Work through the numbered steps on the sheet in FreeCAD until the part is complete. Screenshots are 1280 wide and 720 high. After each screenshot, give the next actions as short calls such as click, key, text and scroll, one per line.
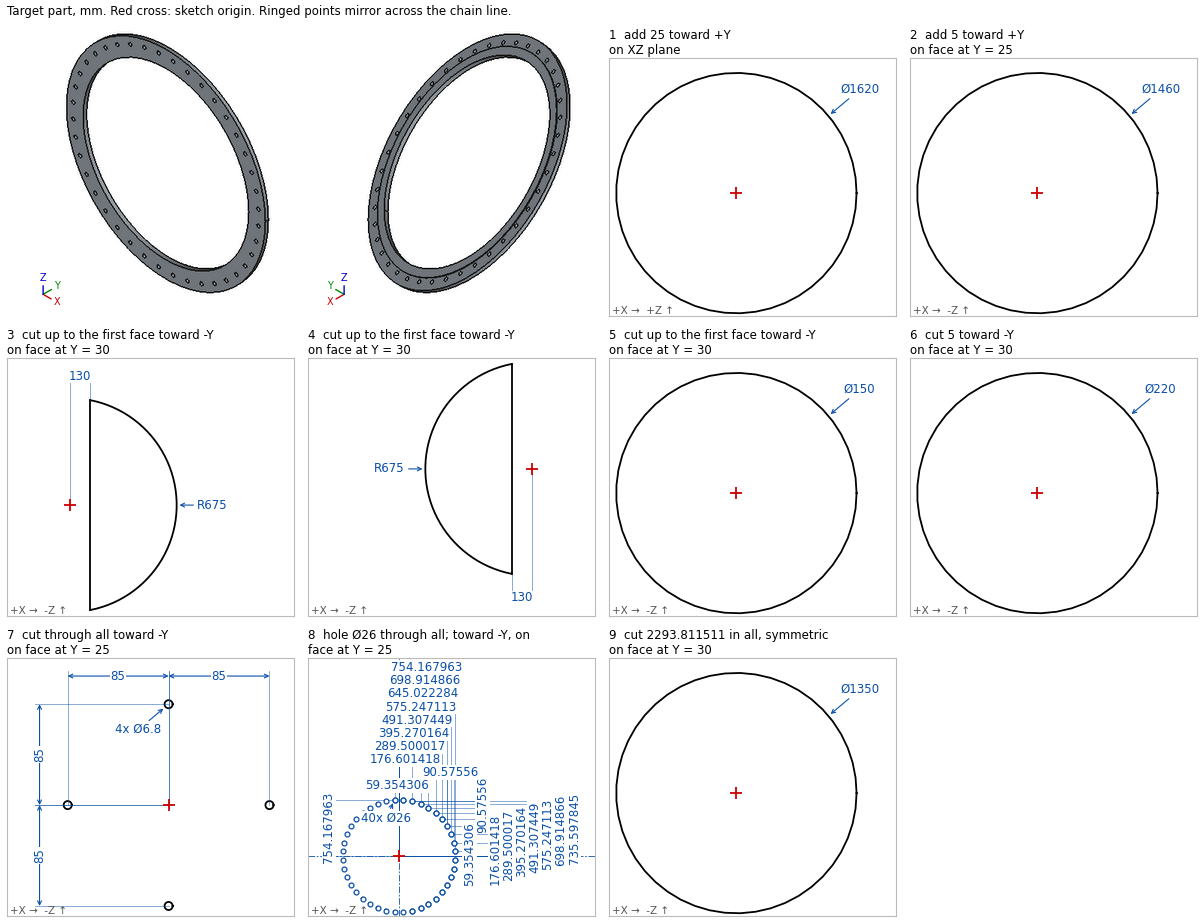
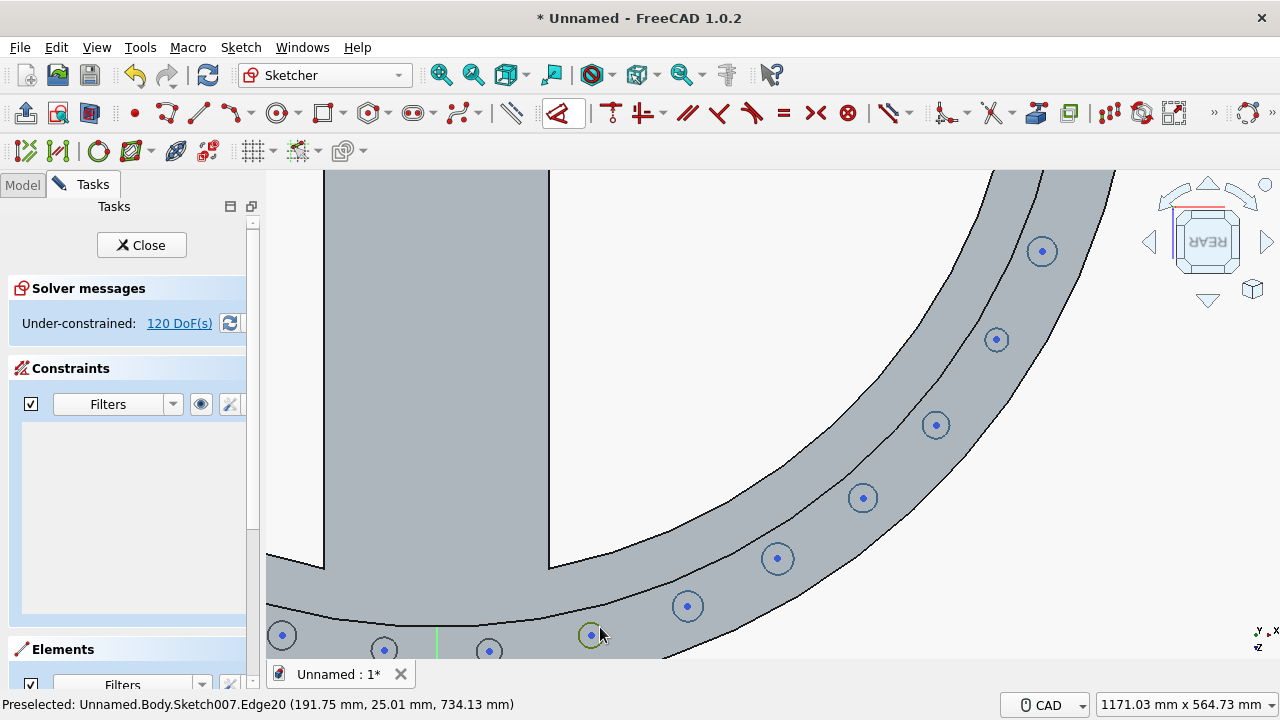
scroll(792, 552, down, 7)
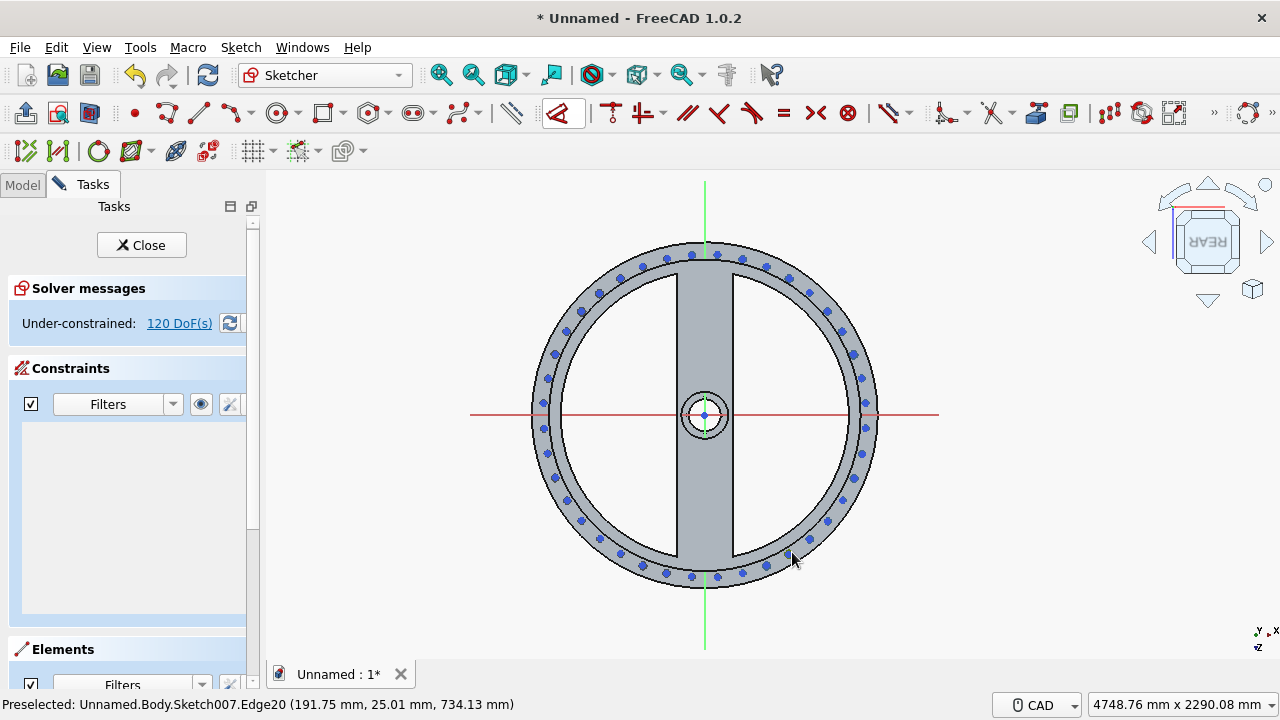
scroll(720, 575, up, 8)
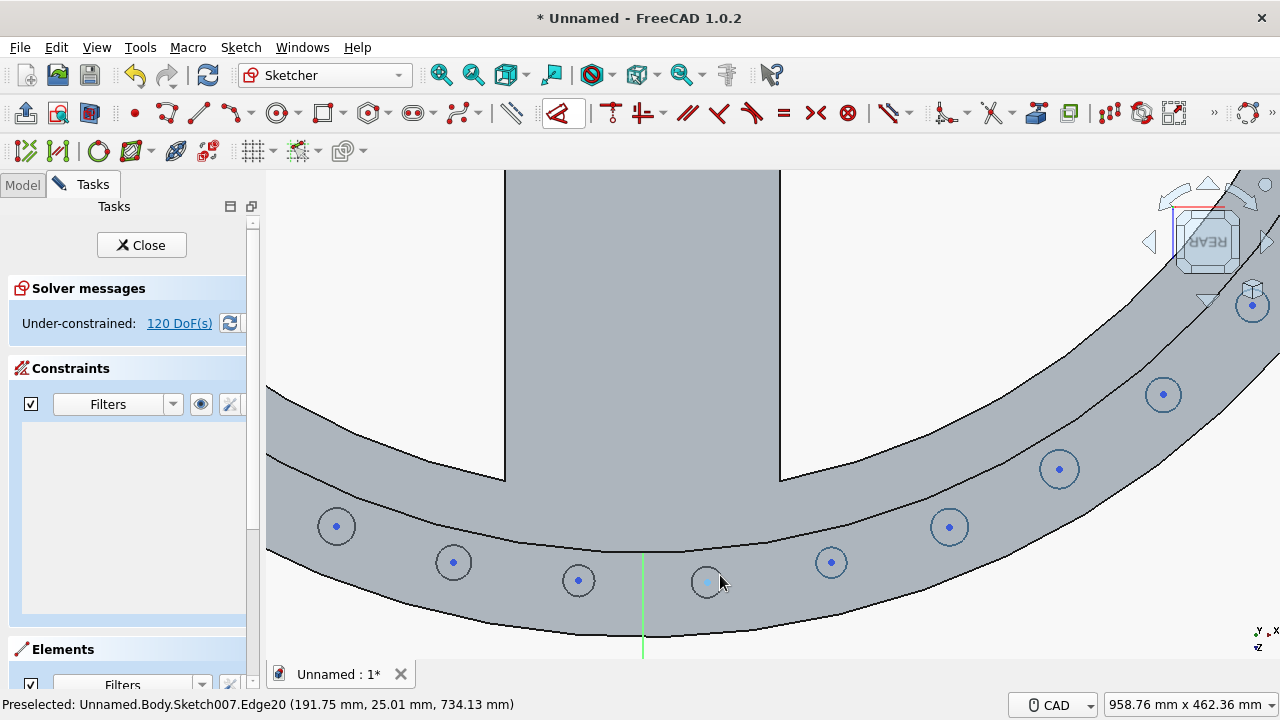
click(718, 571)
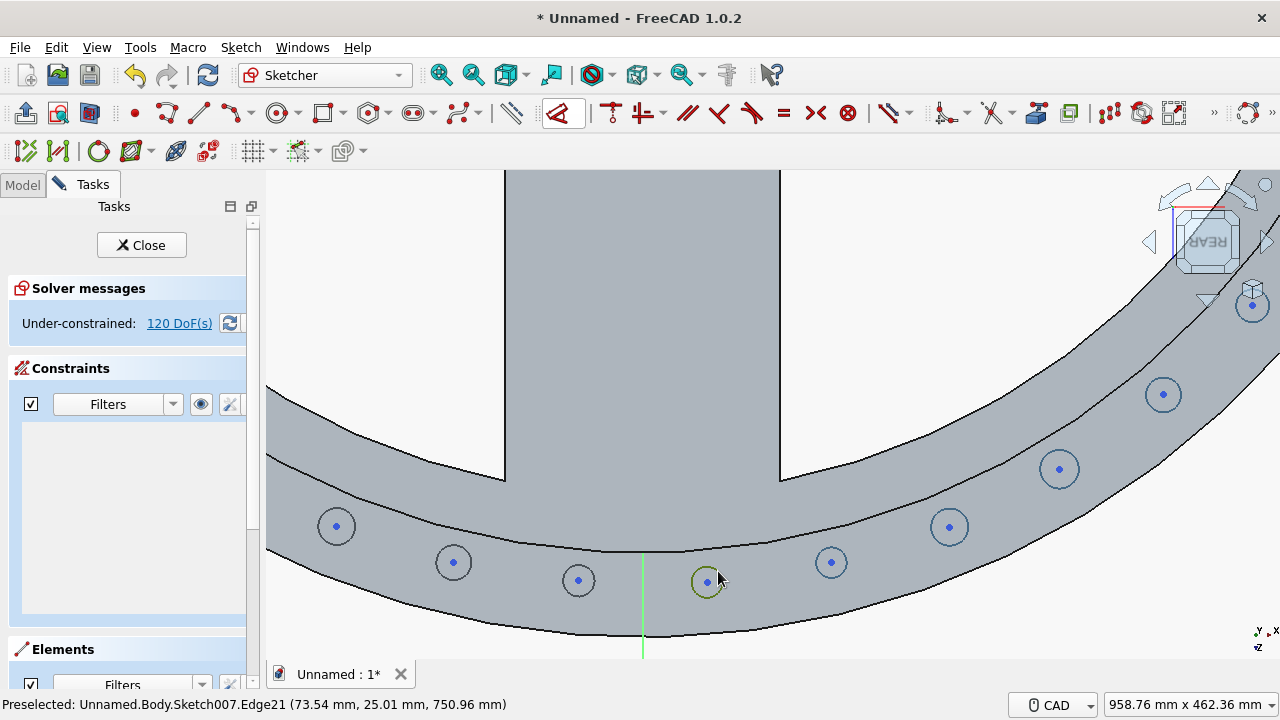
click(590, 570)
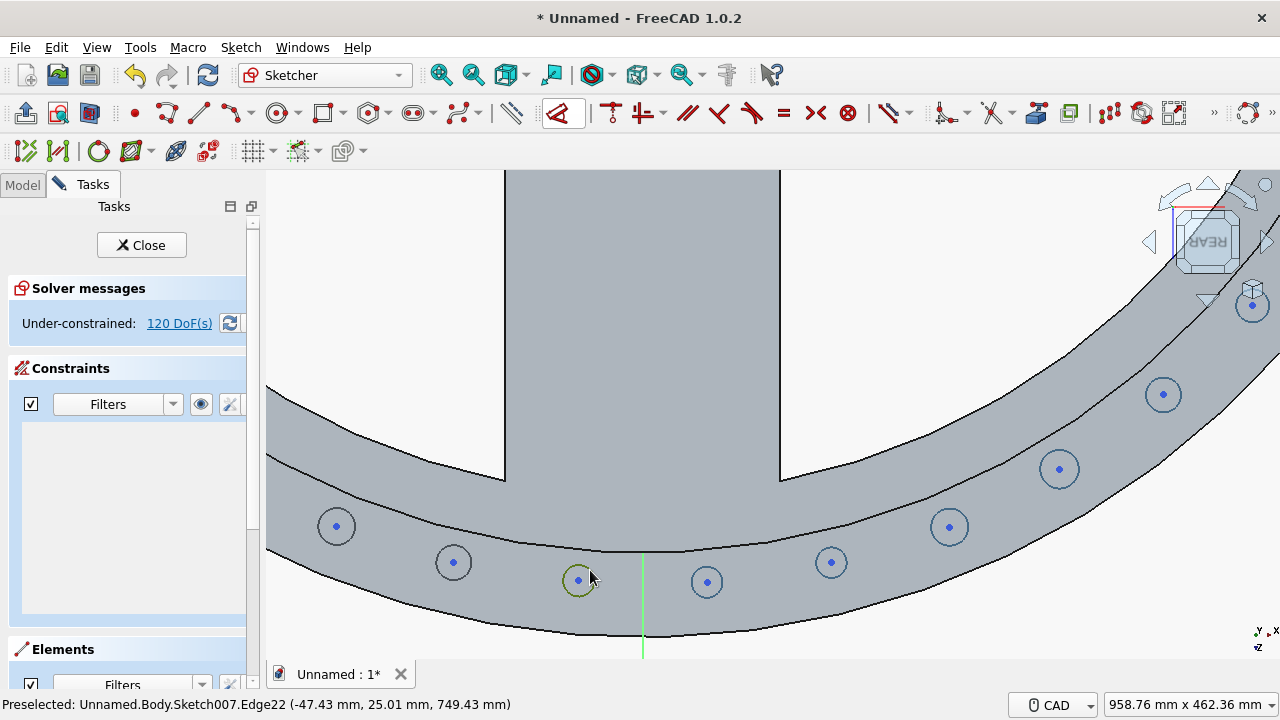
click(466, 550)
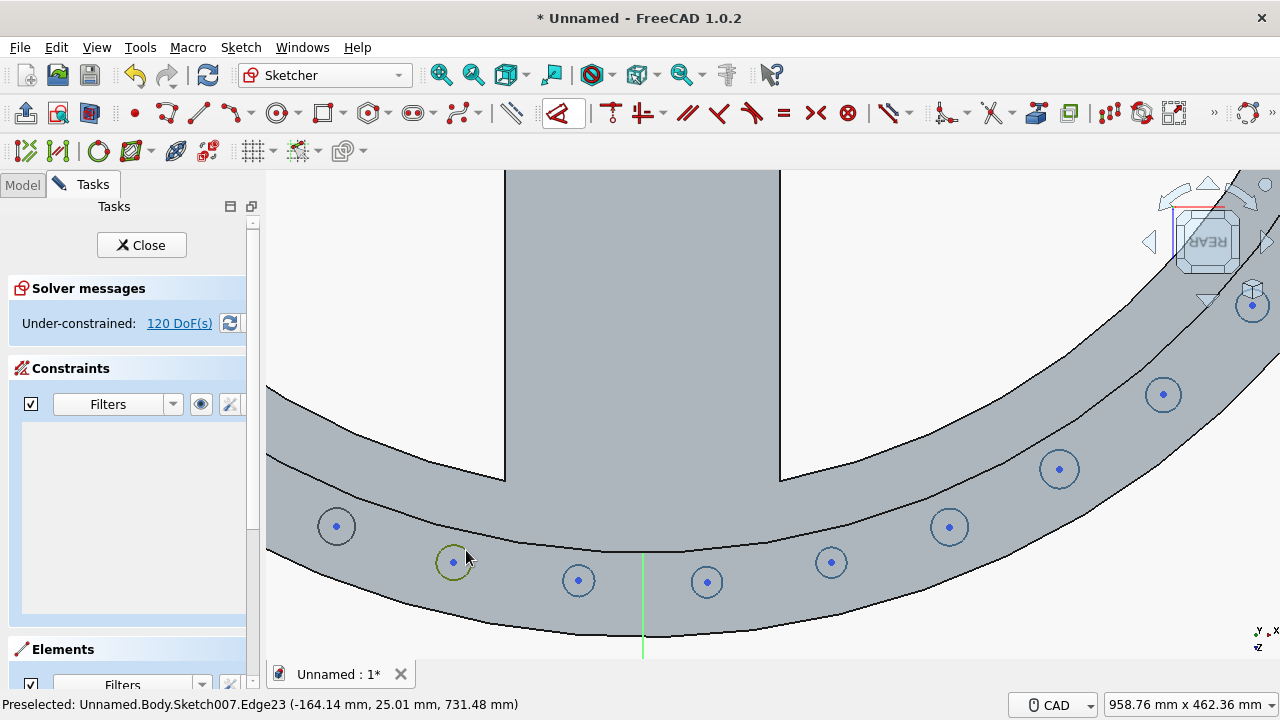
click(350, 513)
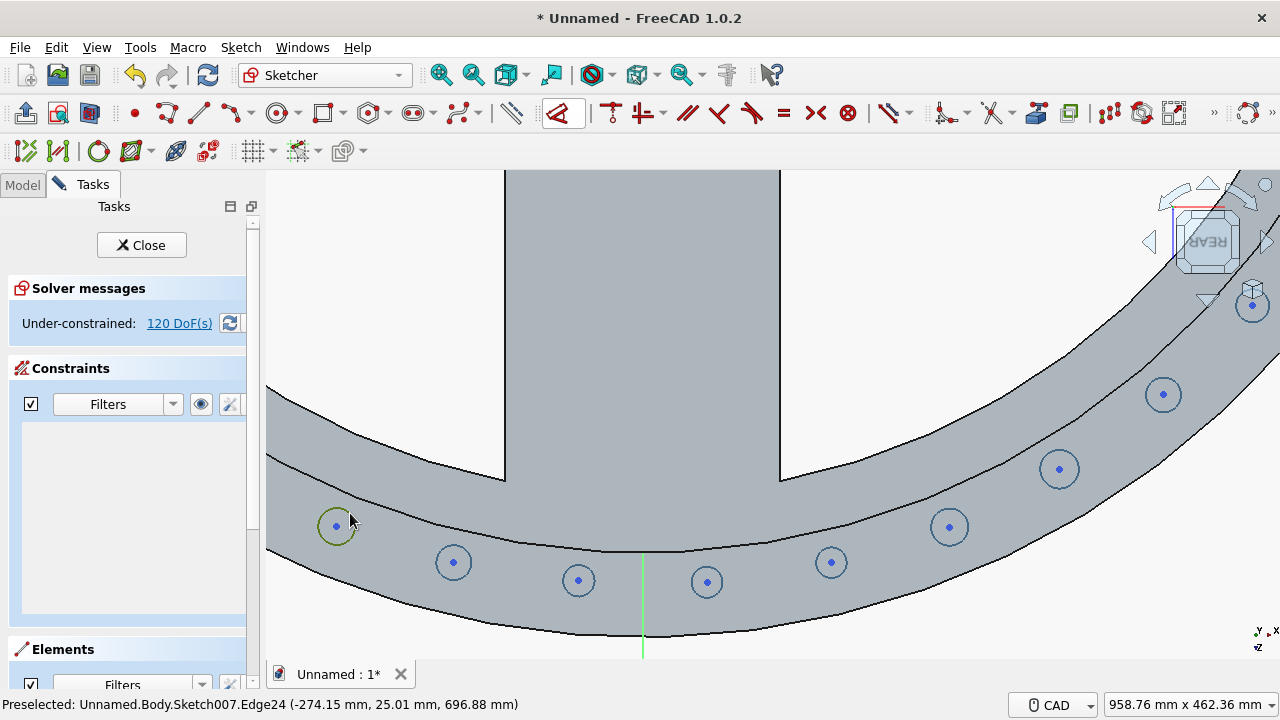
scroll(720, 575, down, 8)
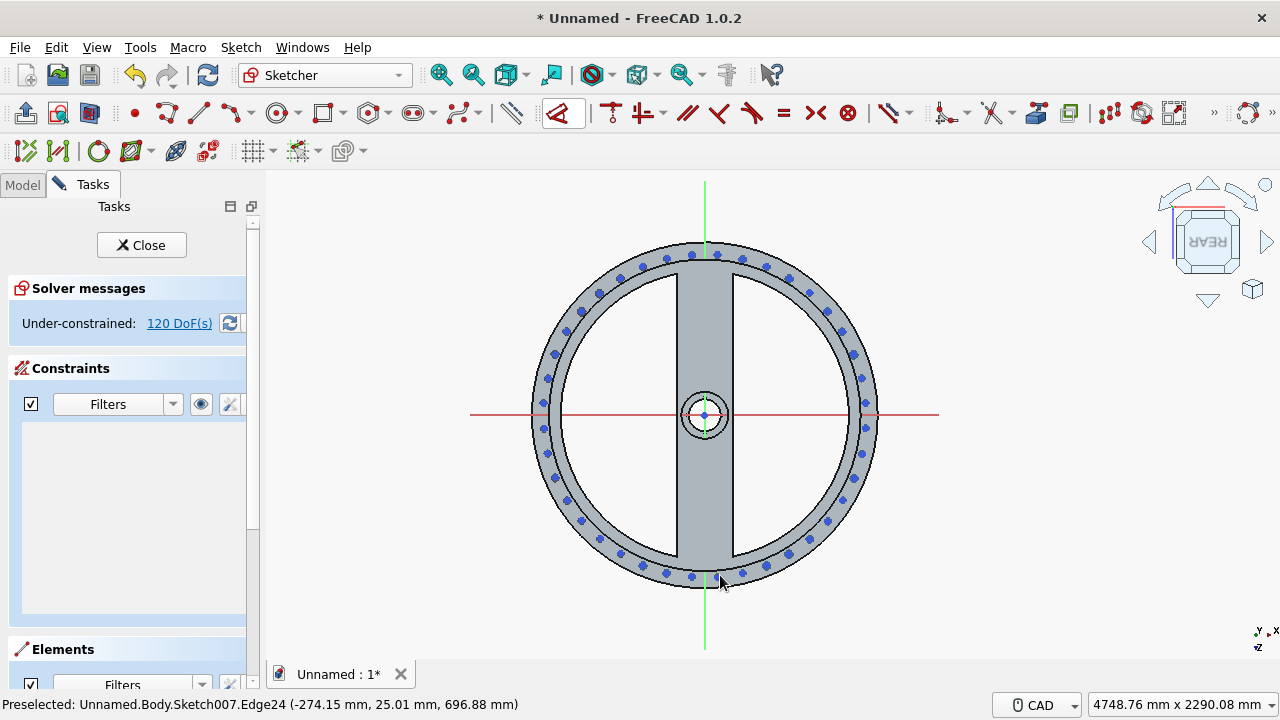
scroll(623, 552, up, 8)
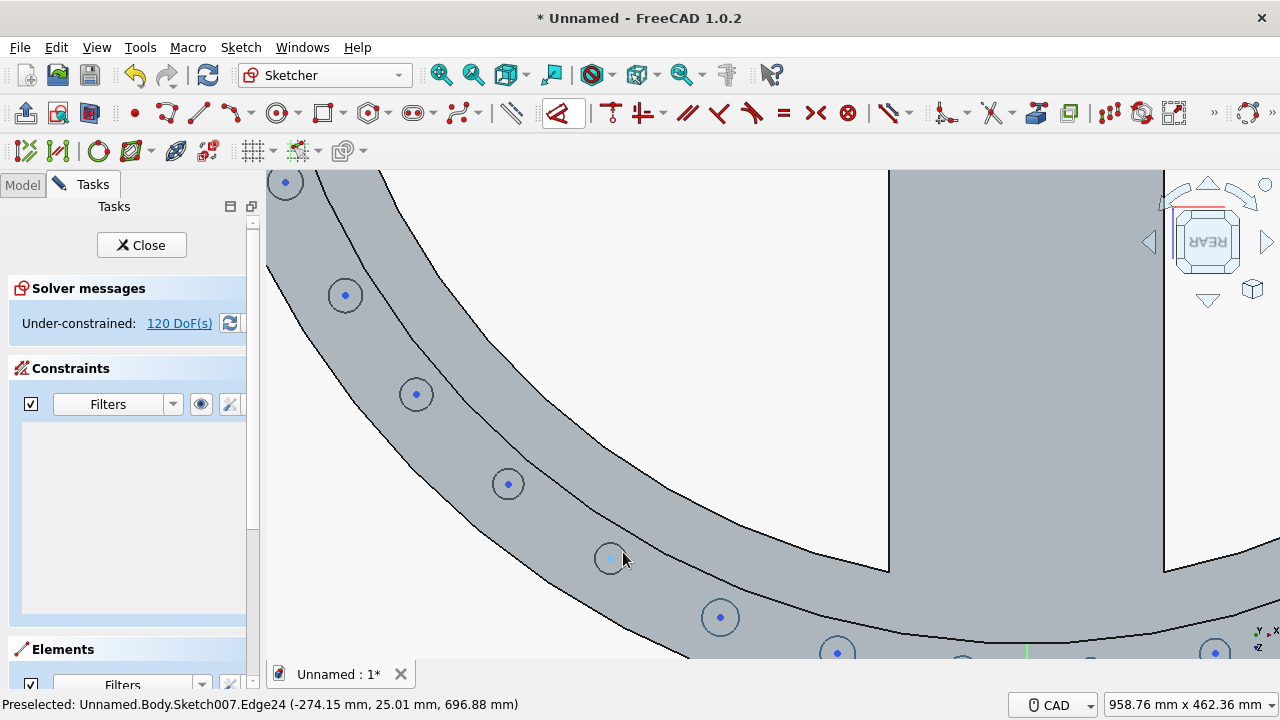
click(621, 548)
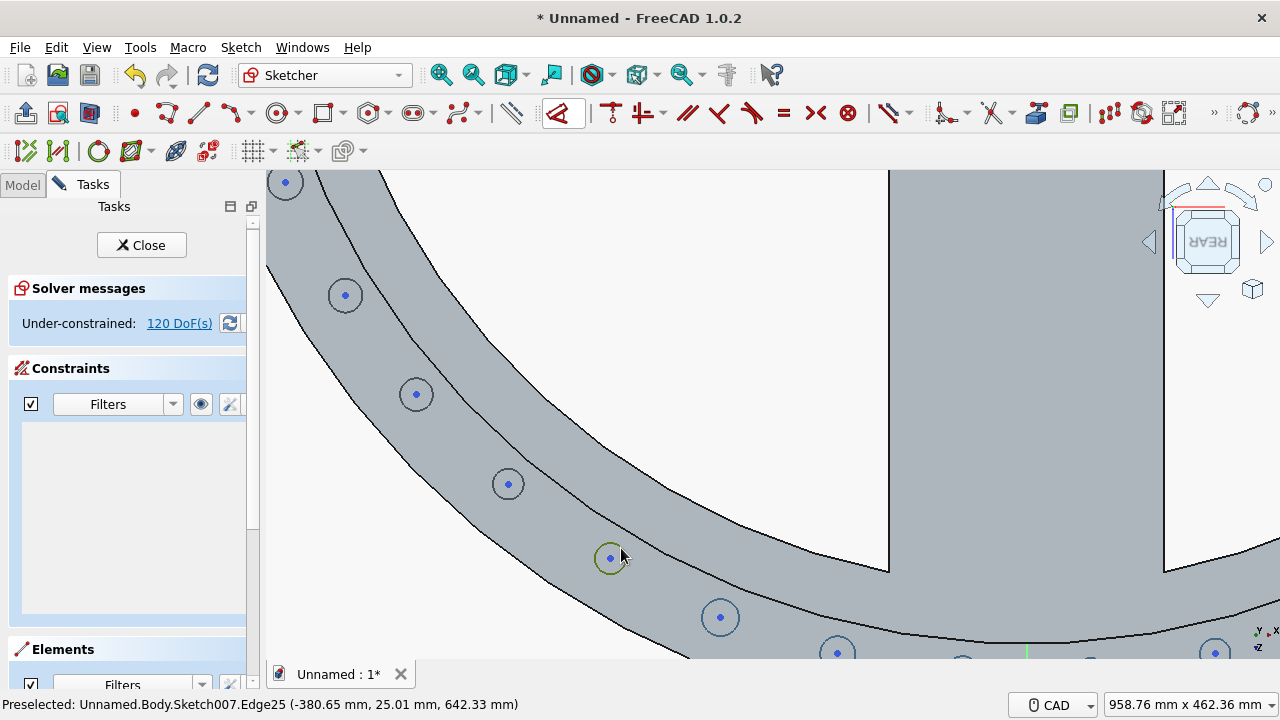
click(519, 473)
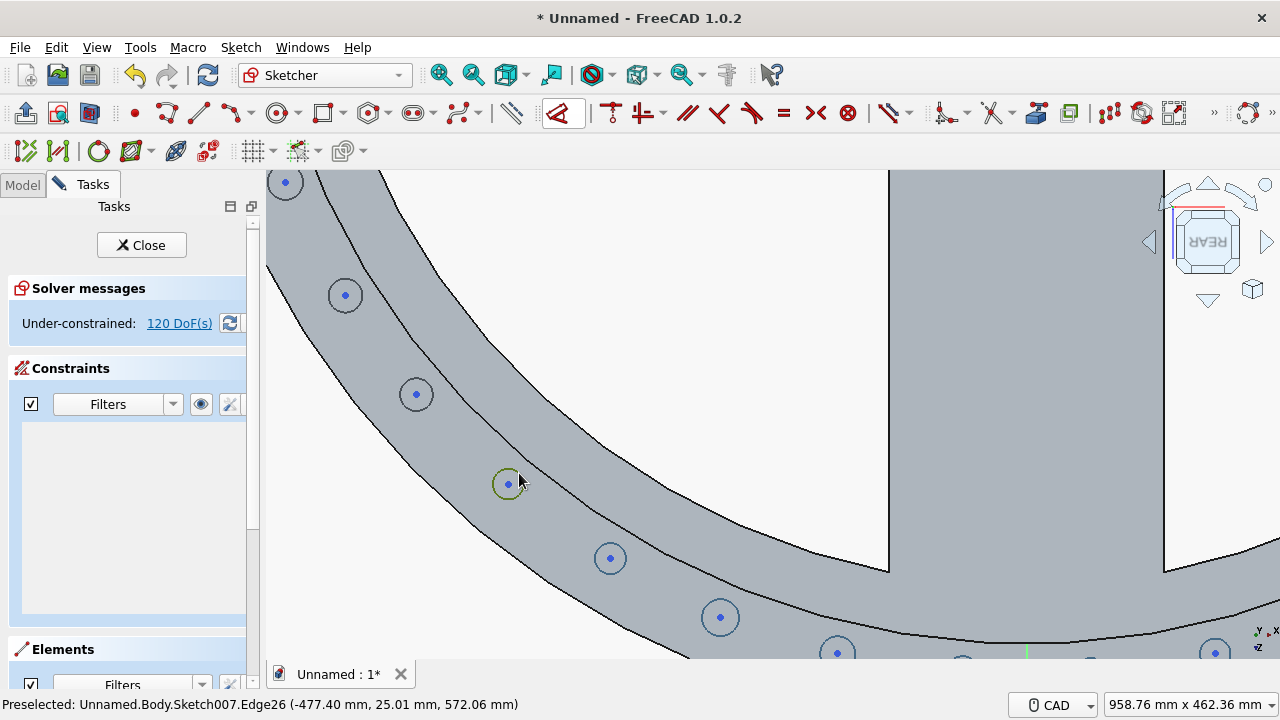
click(428, 383)